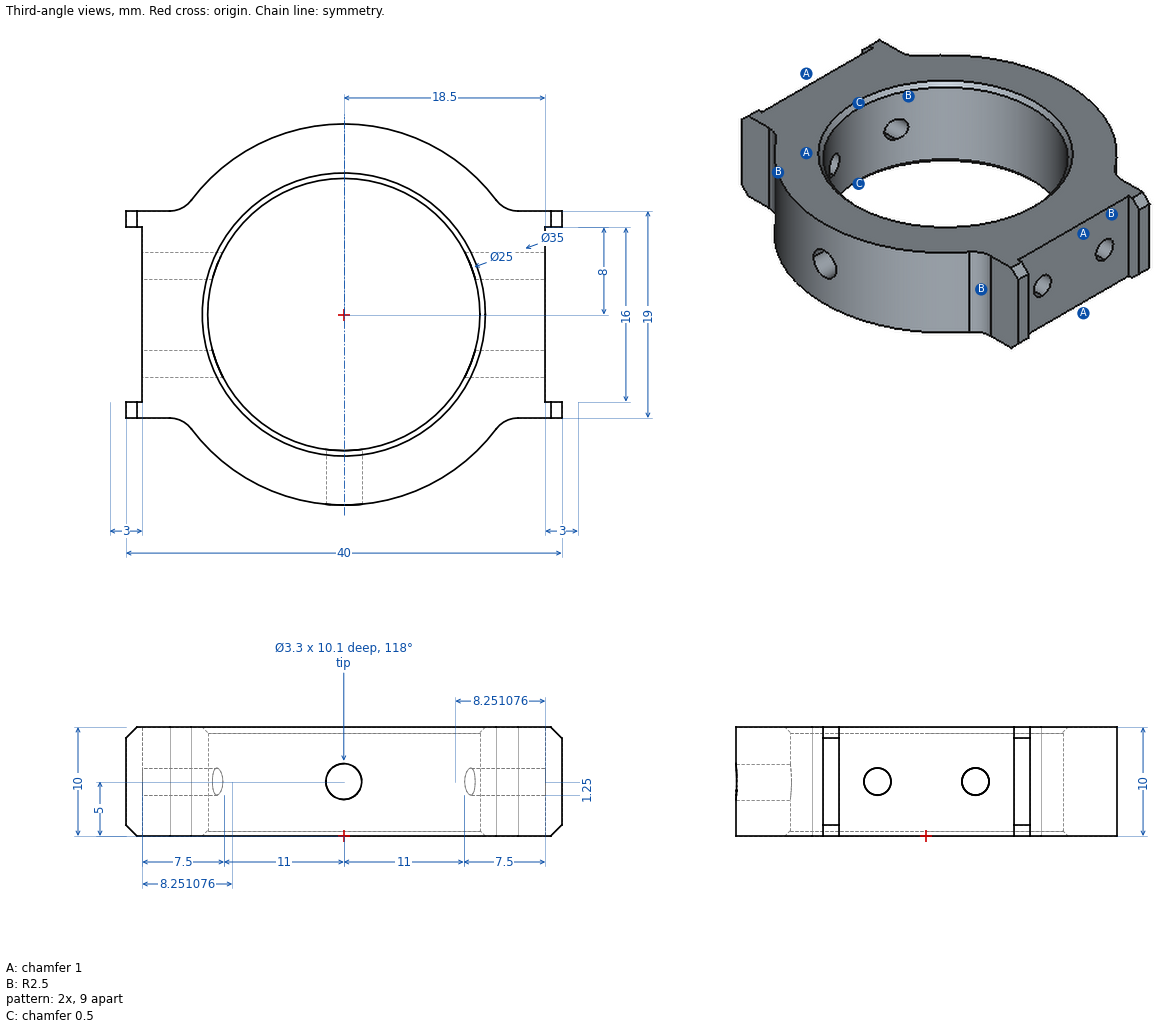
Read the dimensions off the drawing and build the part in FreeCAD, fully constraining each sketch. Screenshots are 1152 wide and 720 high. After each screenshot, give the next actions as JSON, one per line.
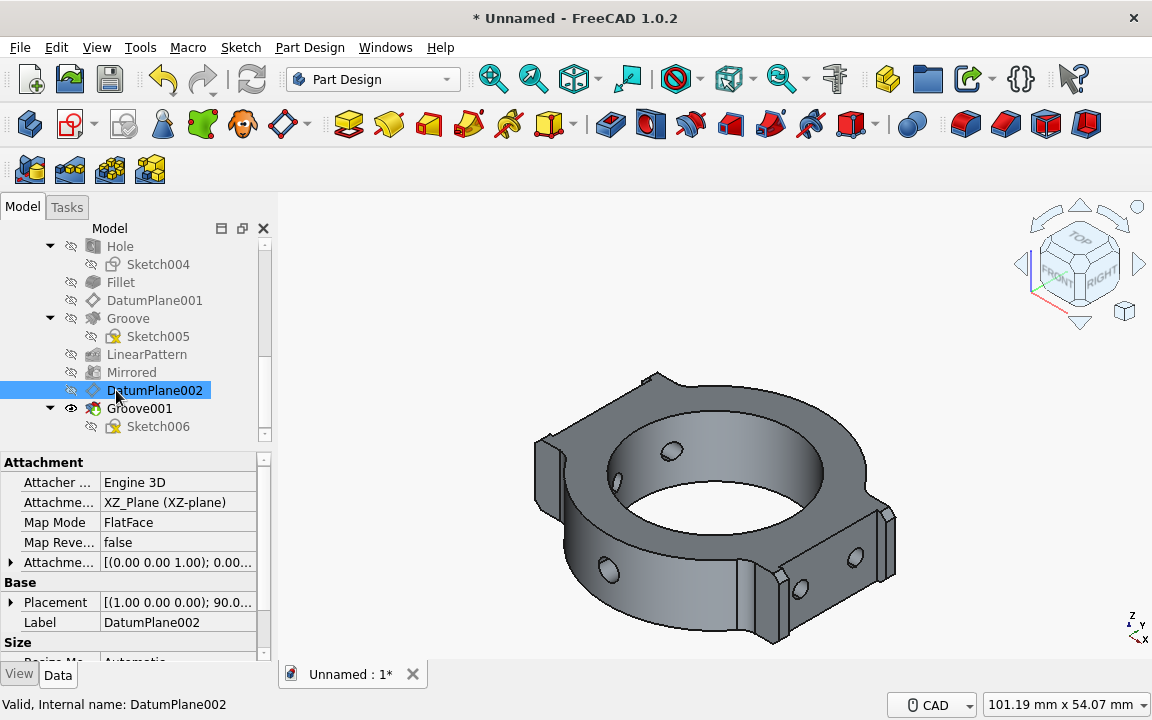
{"action": "left_click", "coordinate": [494, 80]}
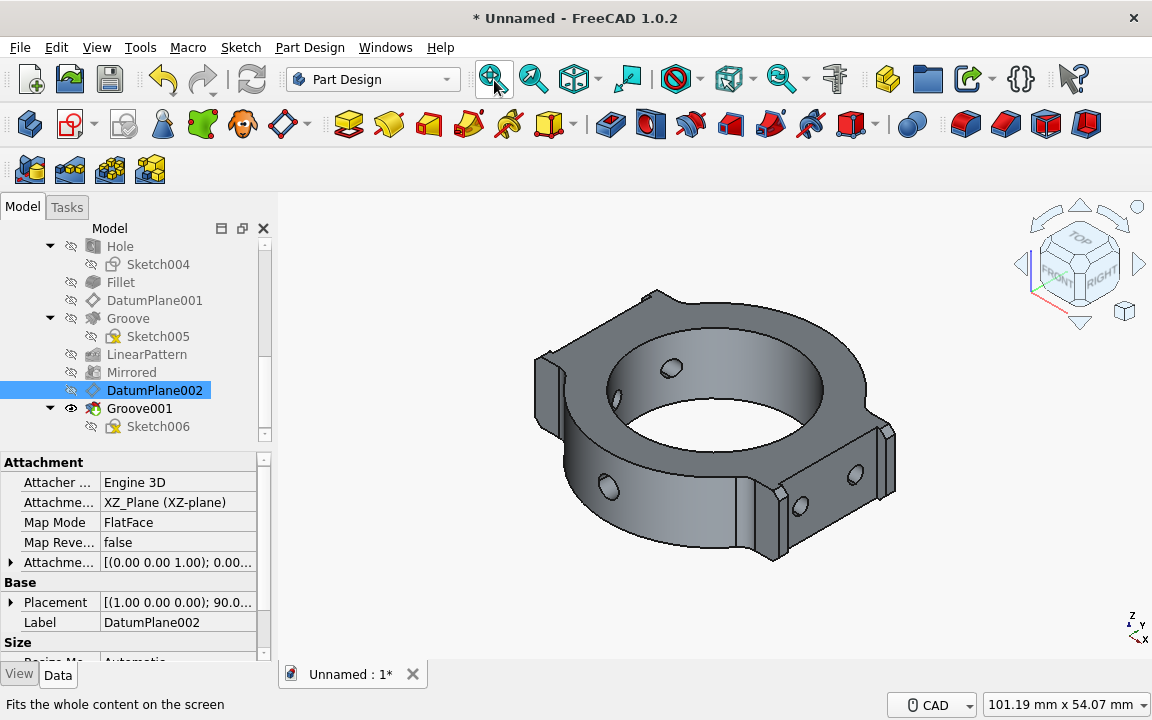
{"action": "left_click", "coordinate": [639, 345]}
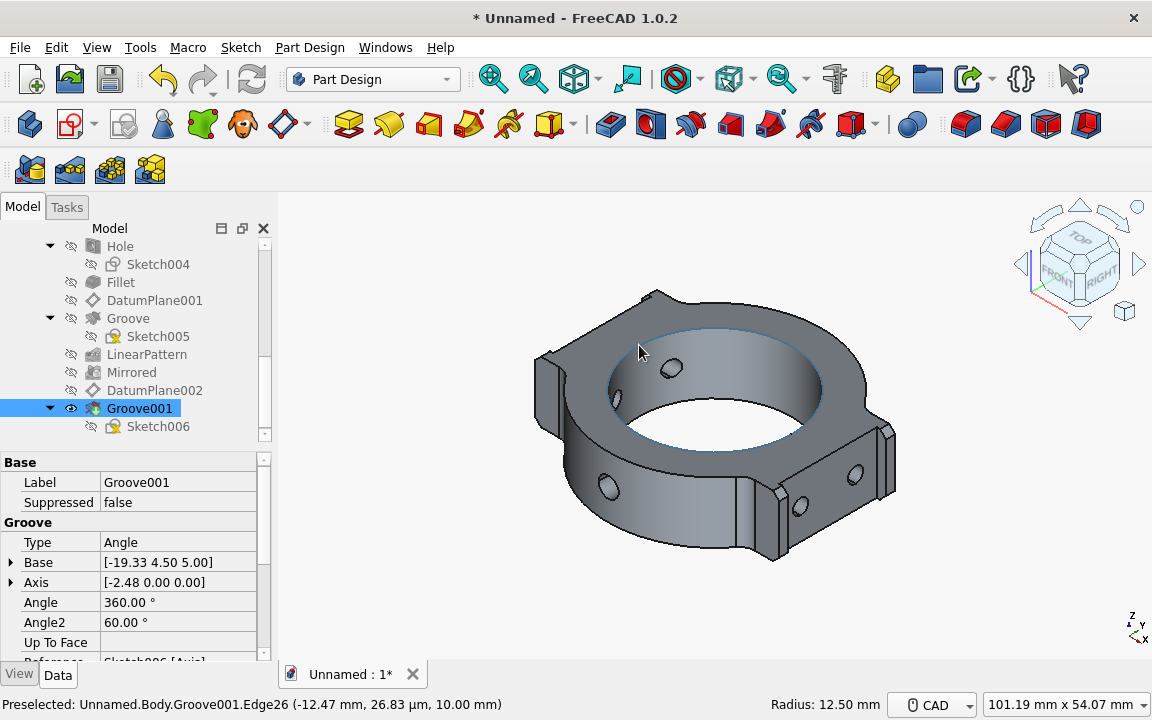
{"action": "key", "text": "2"}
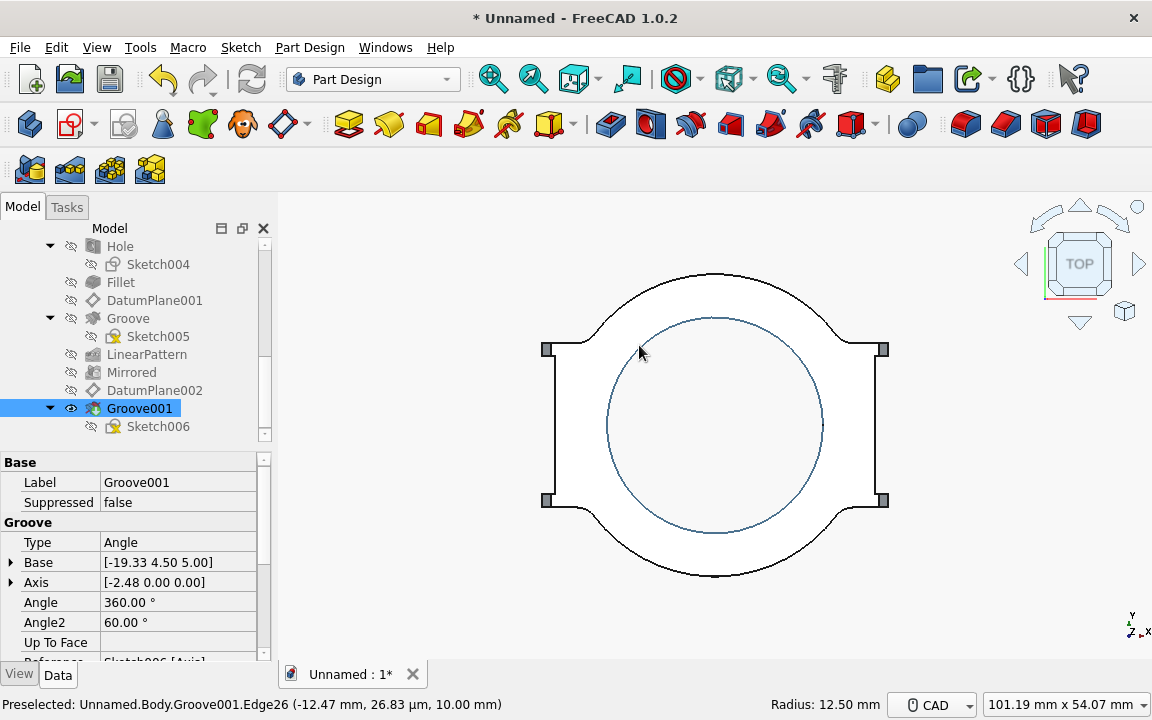
{"action": "key", "text": "0"}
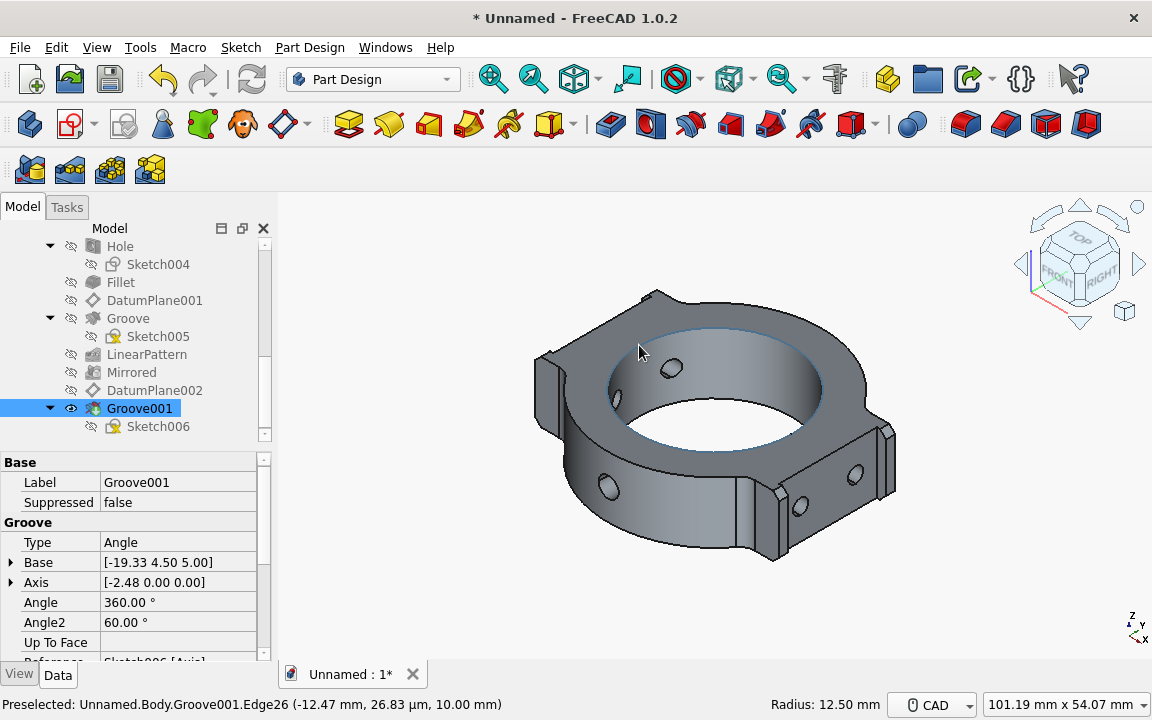
{"action": "key", "text": "1"}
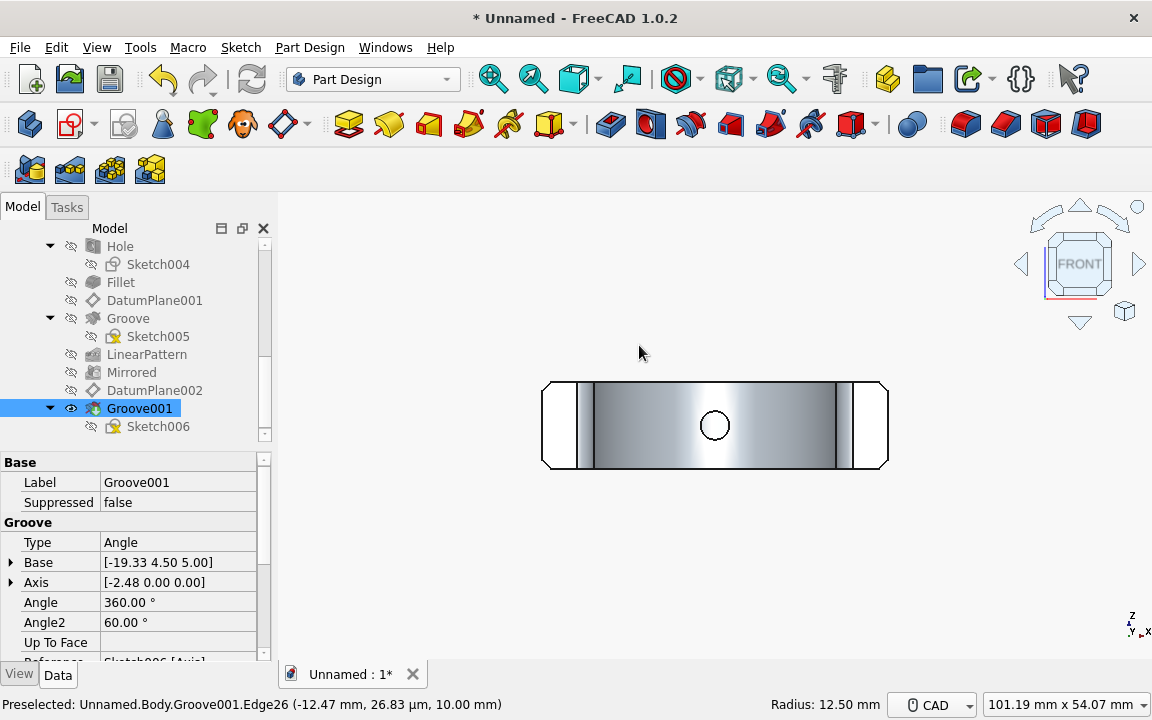
{"action": "left_click", "coordinate": [494, 80]}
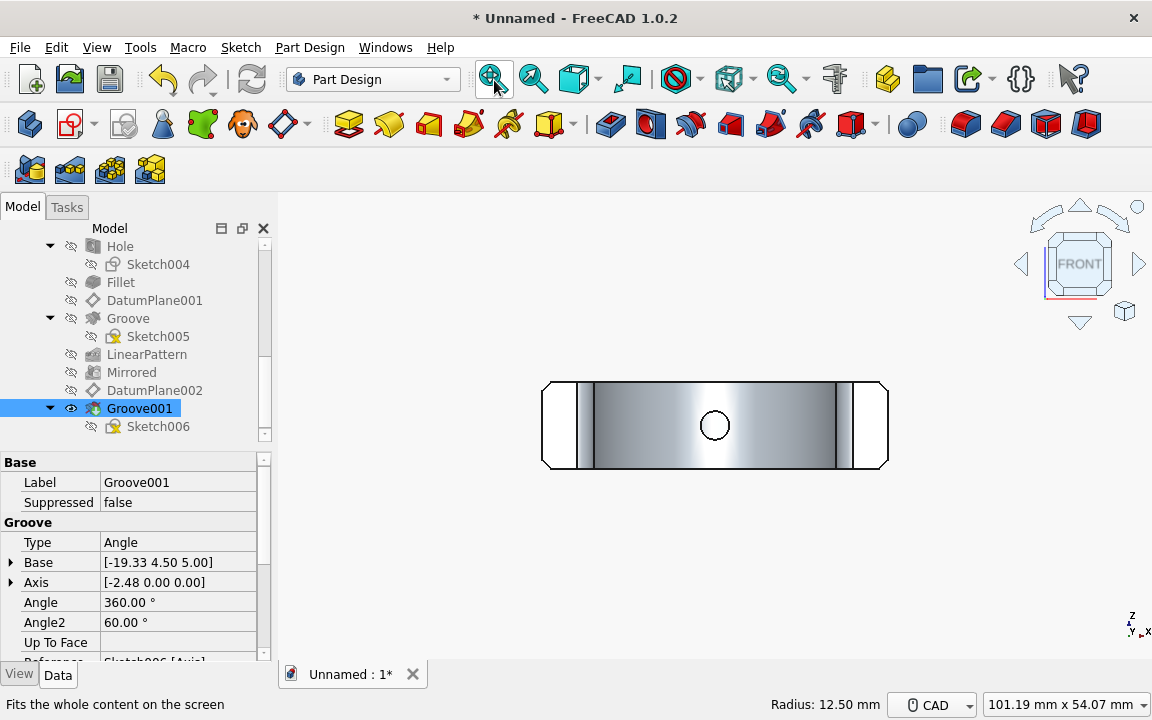
{"action": "key", "text": "3"}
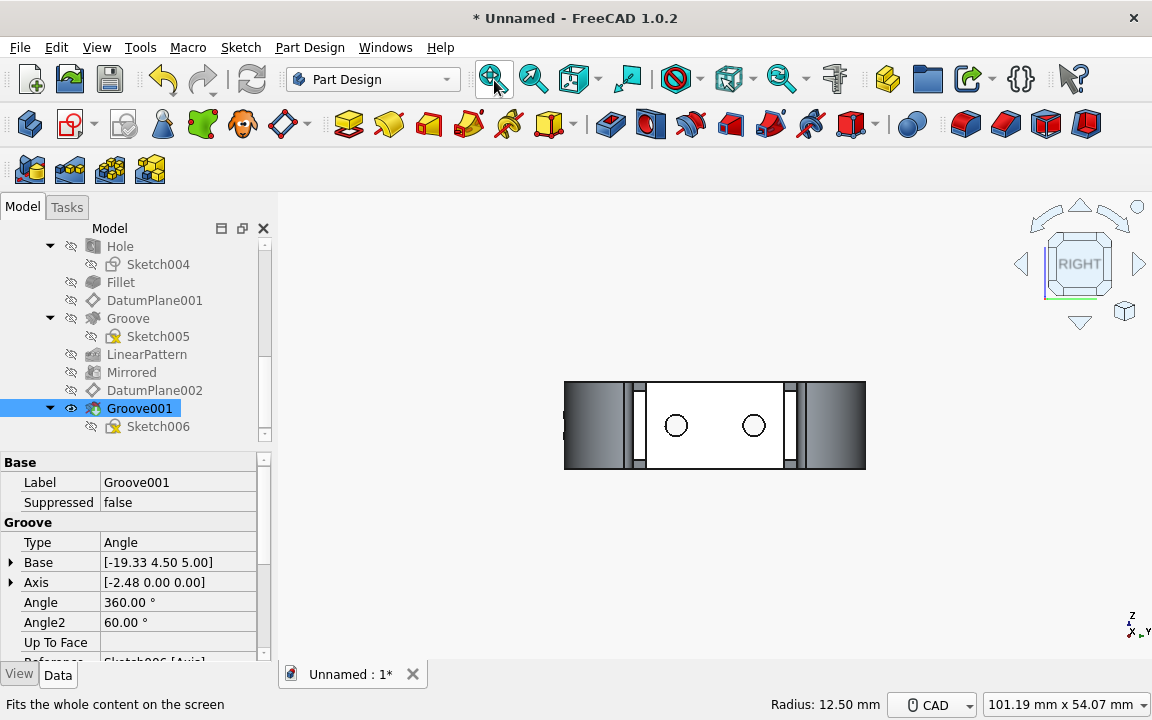
{"action": "key", "text": "v f"}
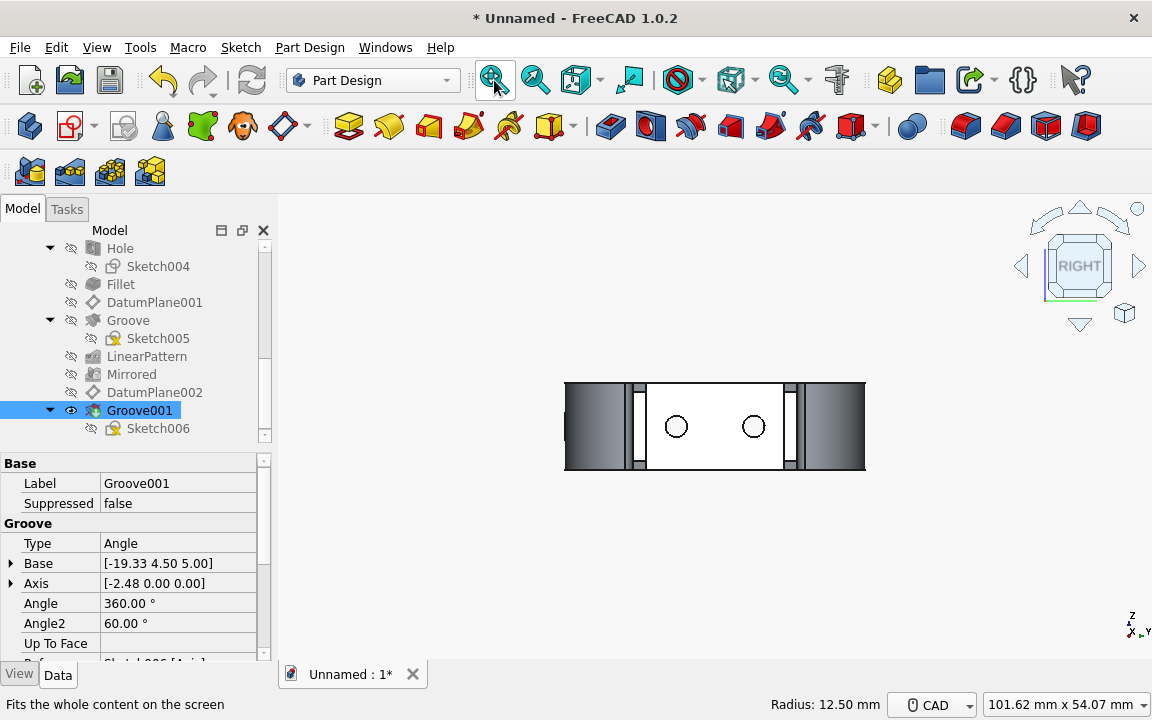
{"action": "key", "text": "5"}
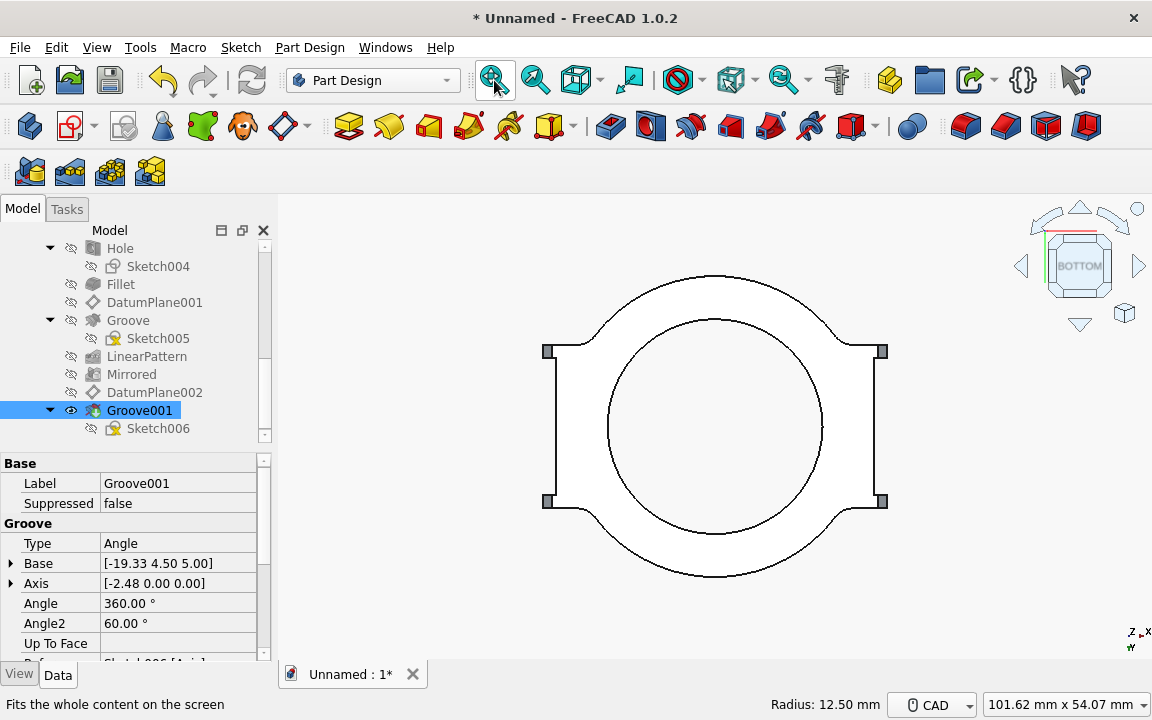
{"action": "left_click", "coordinate": [607, 426], "text": "ctrl"}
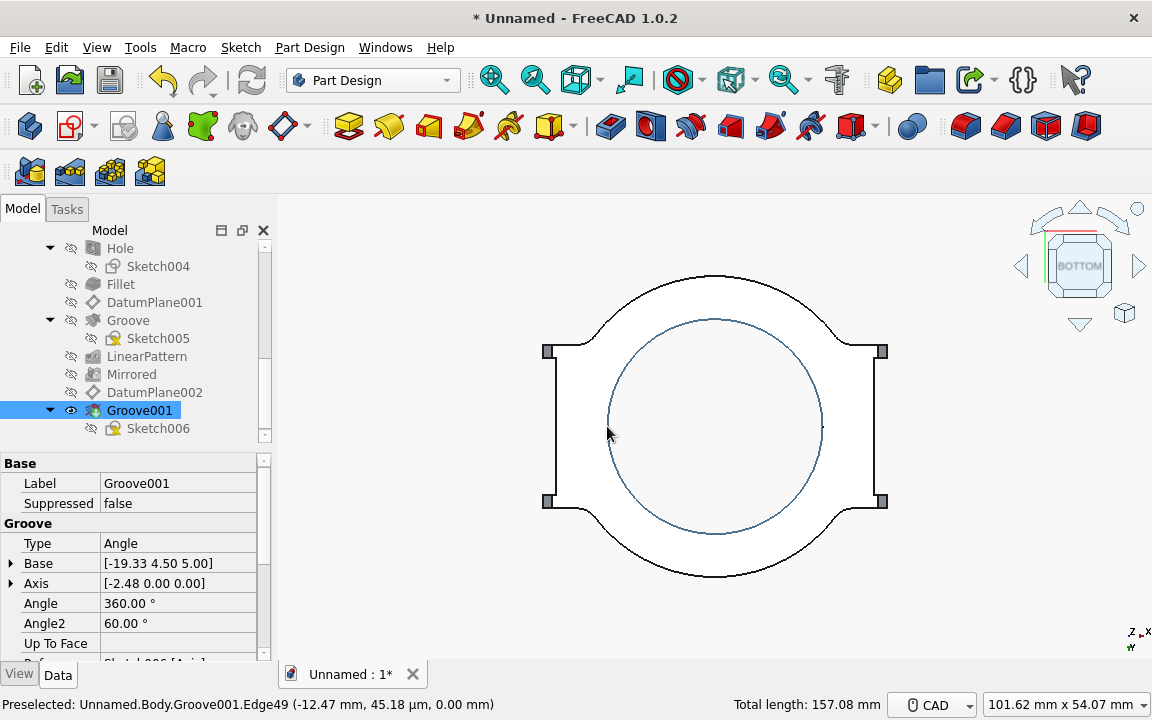
{"action": "left_click", "coordinate": [1006, 126]}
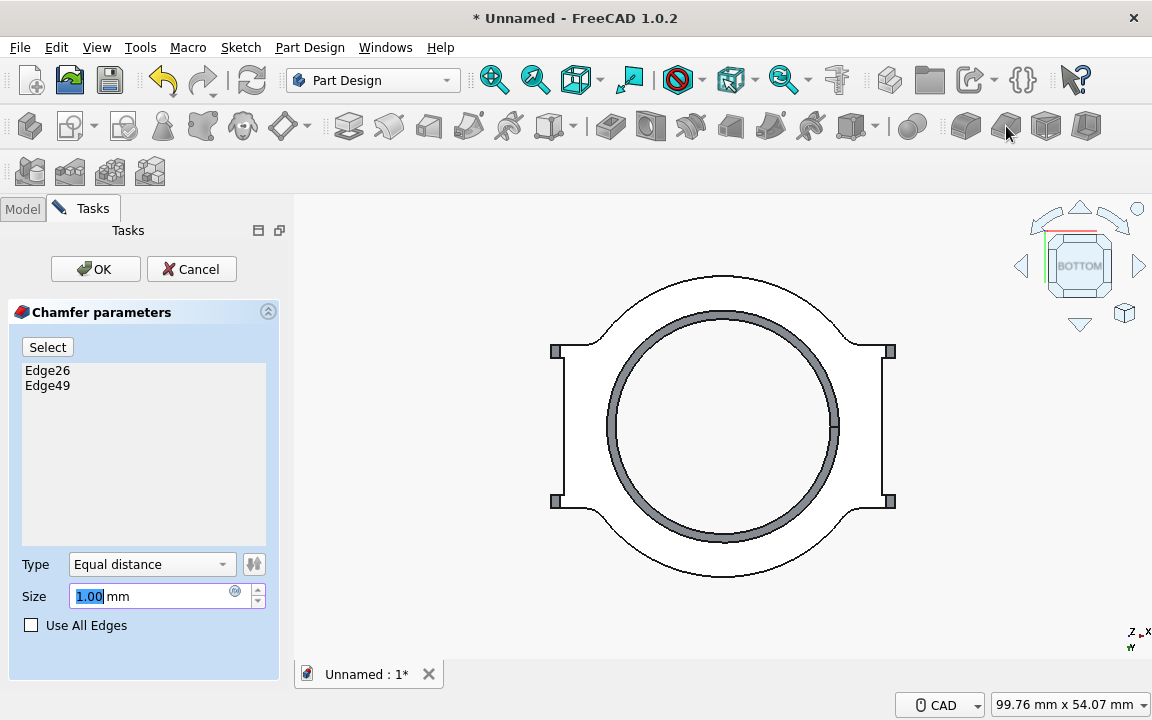
{"action": "type", "text": "0.5"}
{"action": "key", "text": "Tab"}